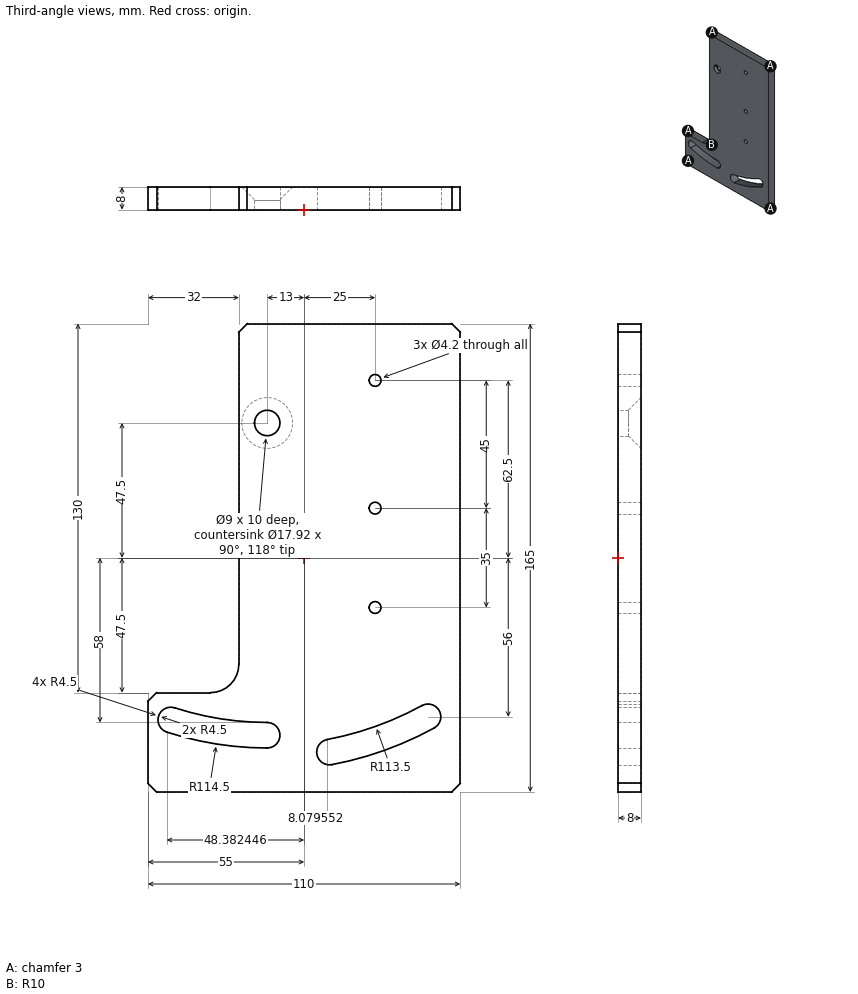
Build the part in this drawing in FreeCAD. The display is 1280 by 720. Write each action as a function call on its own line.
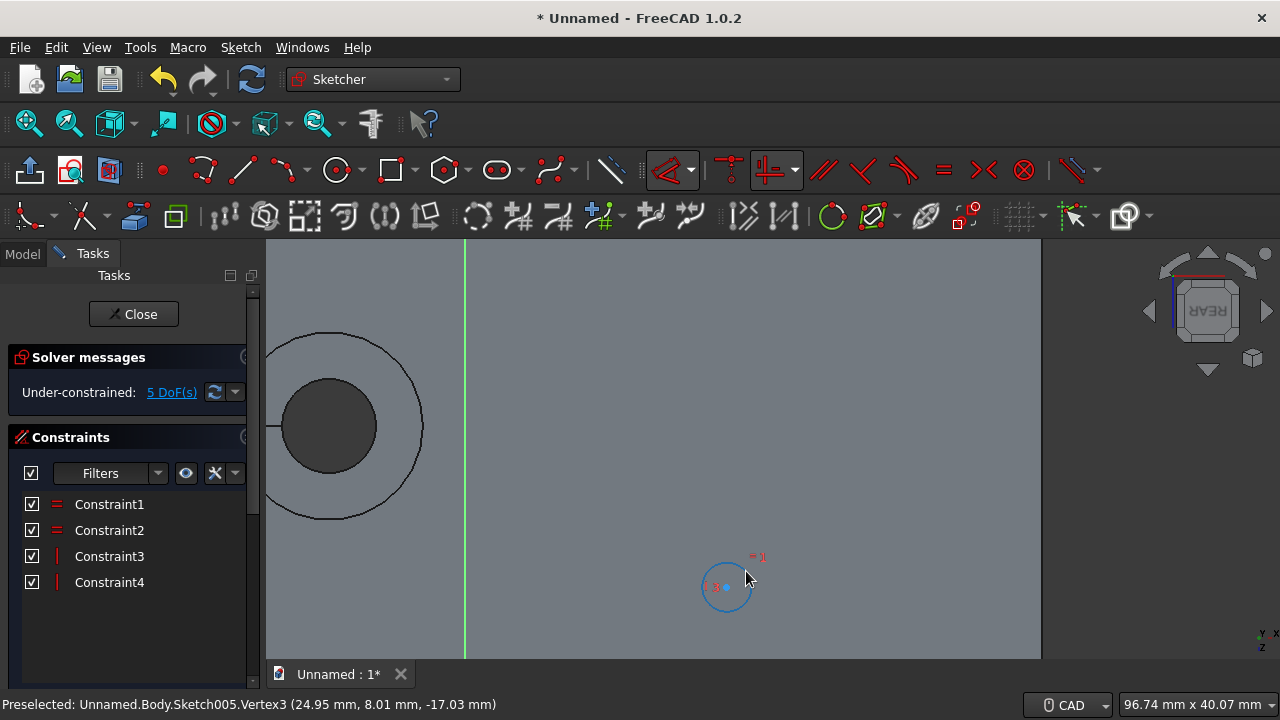
click(744, 570)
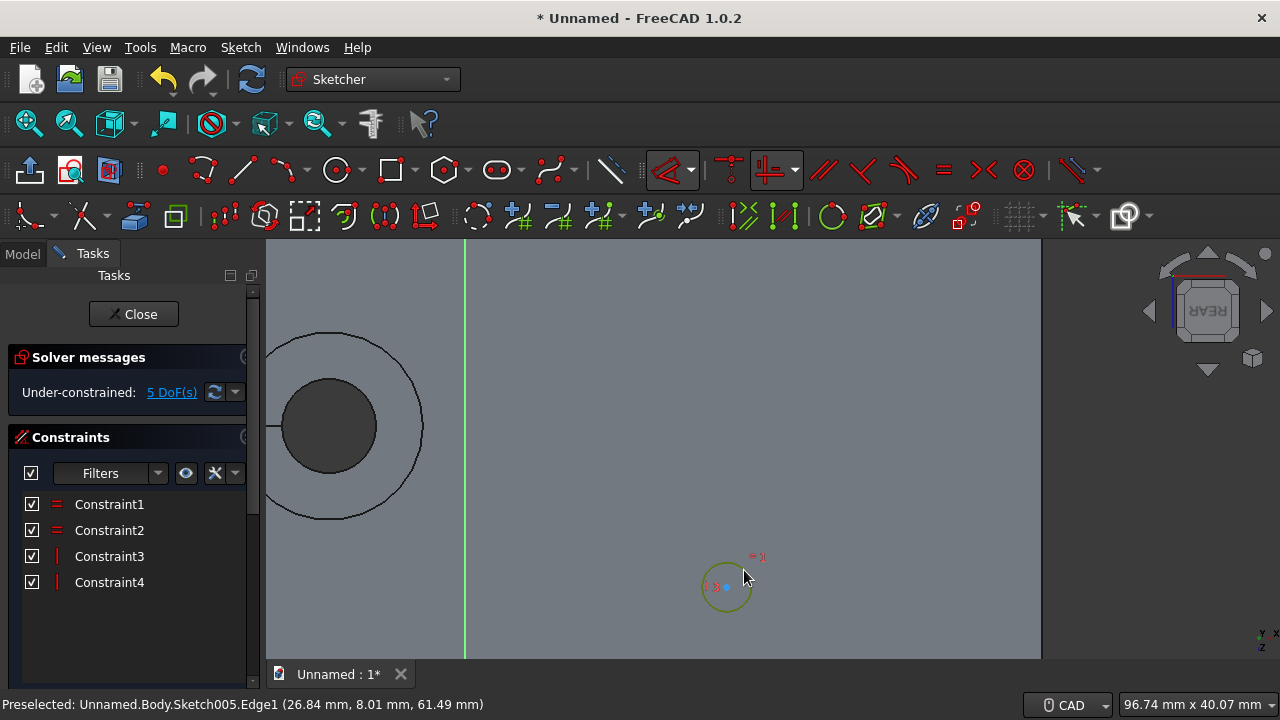
click(694, 170)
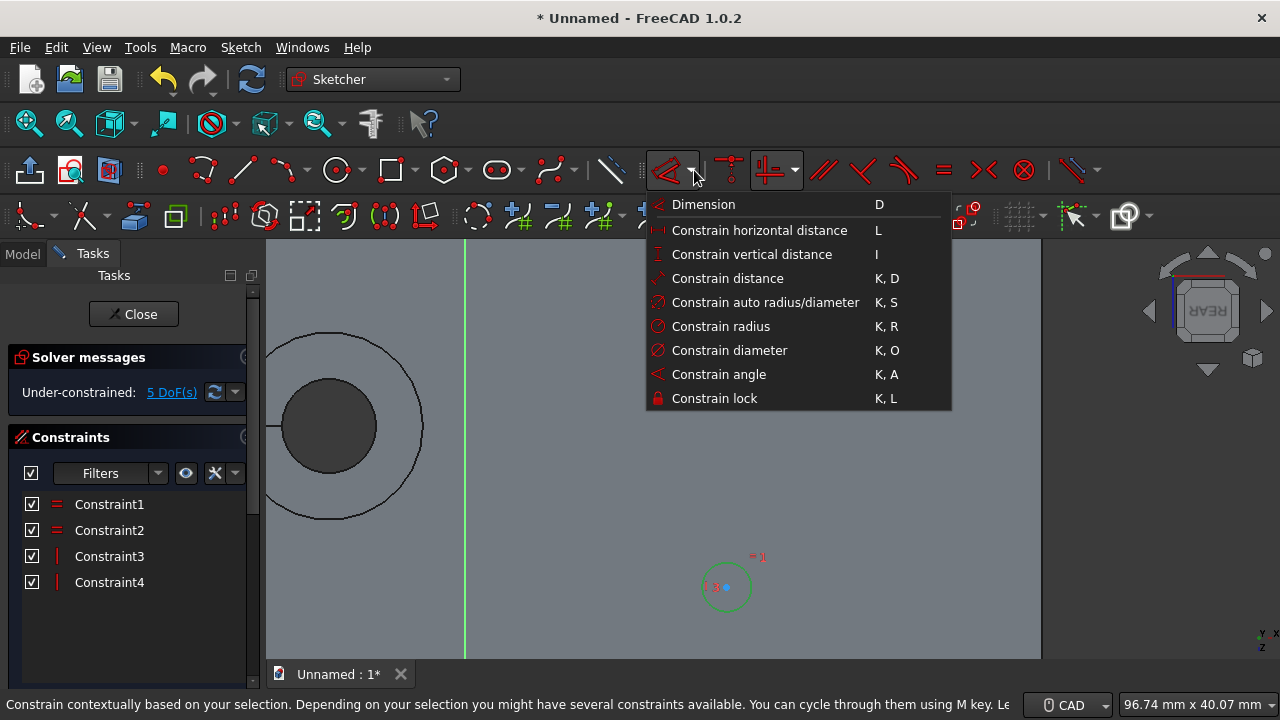
click(799, 350)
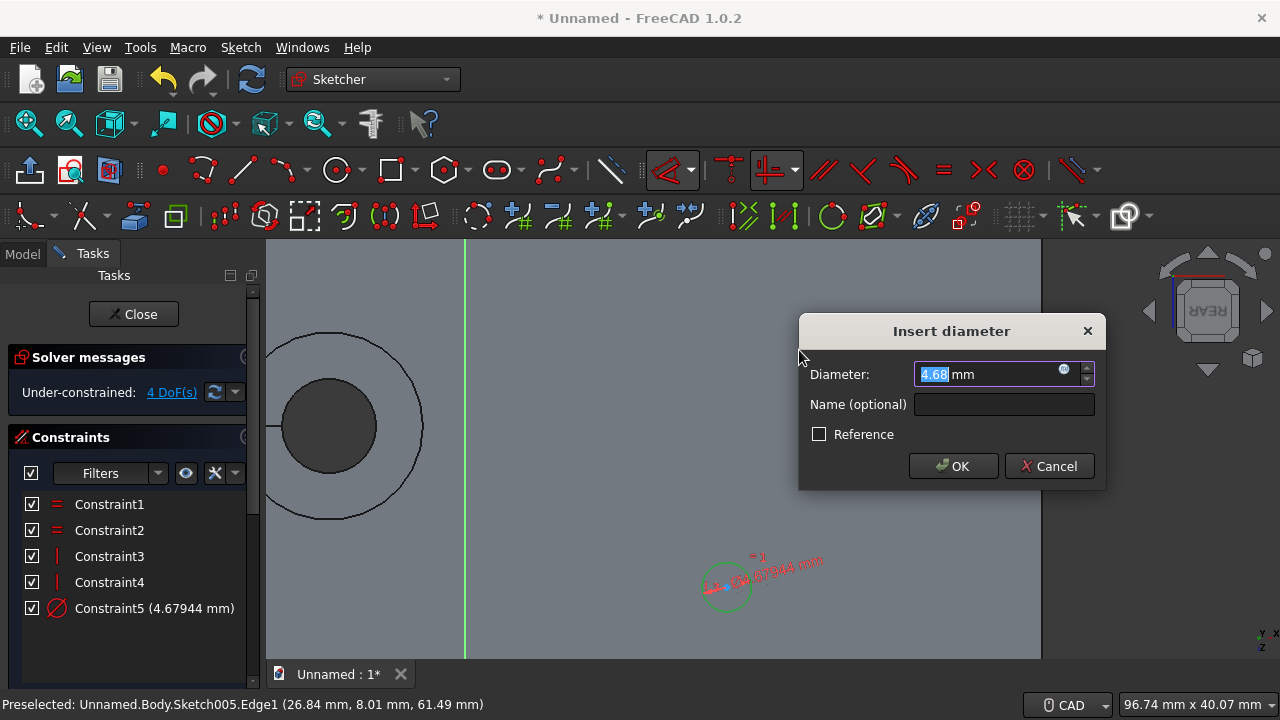
text(4.2)
key(Return)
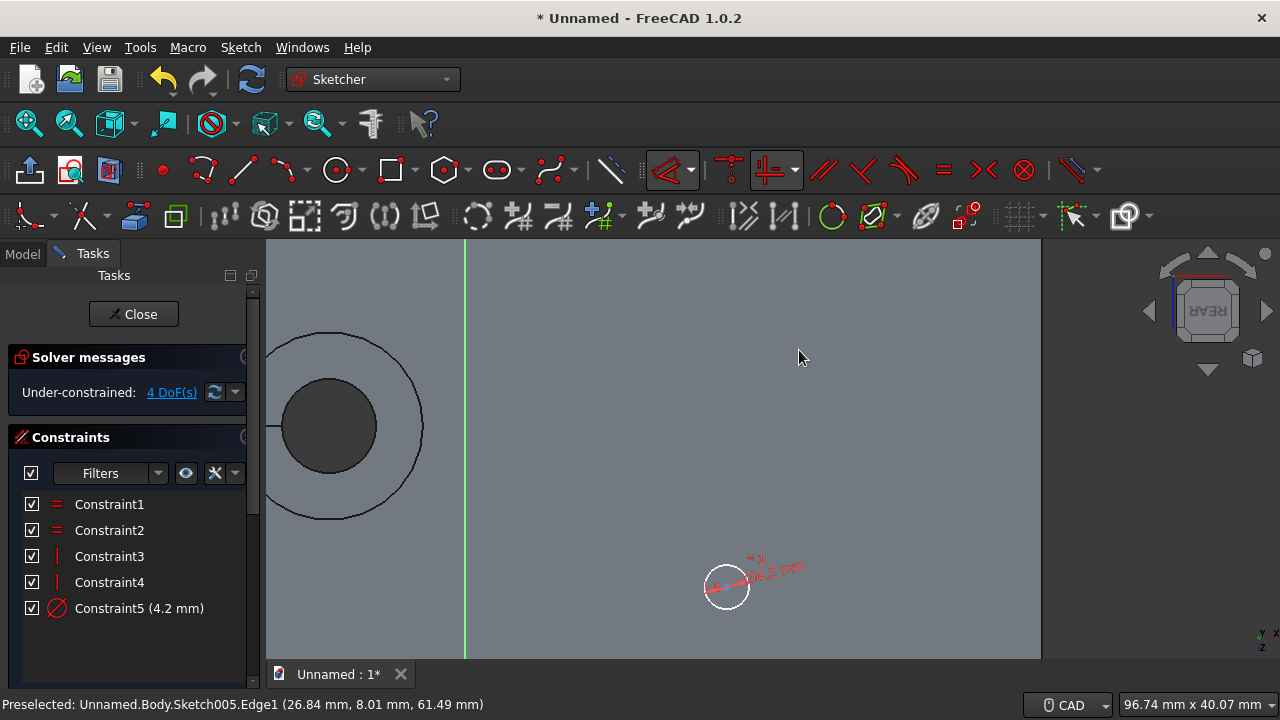
click(727, 587)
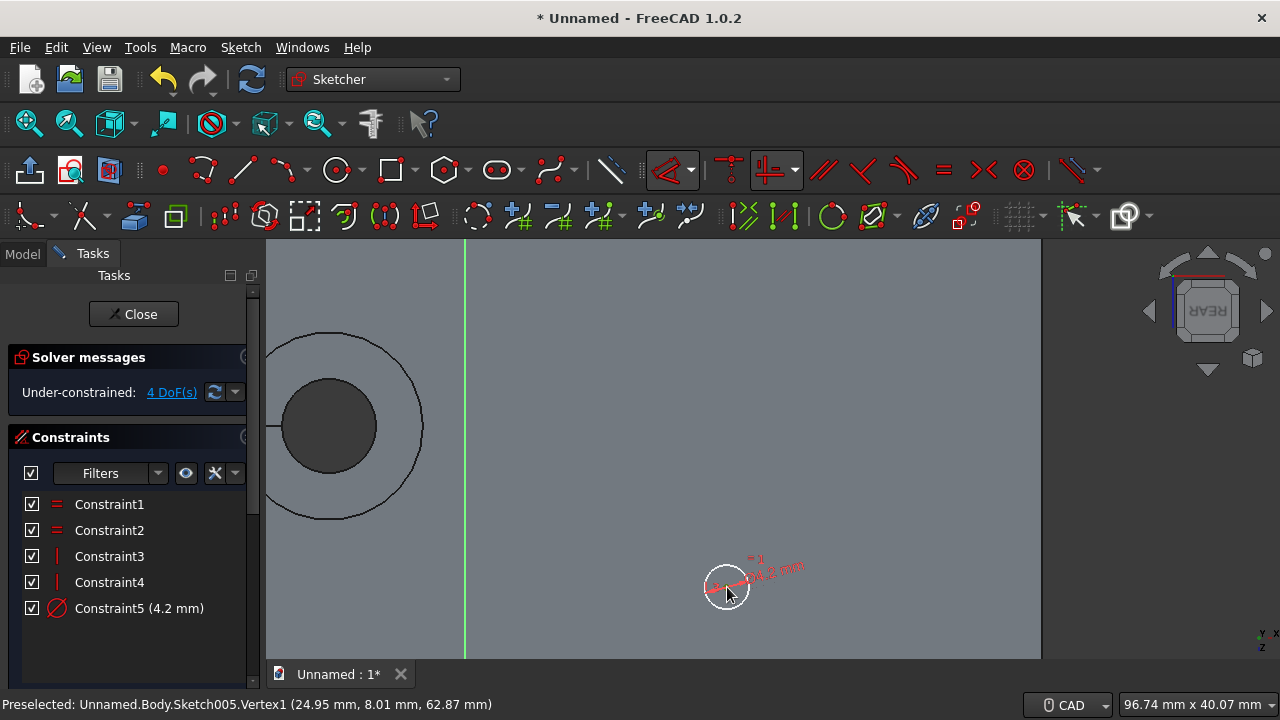
click(694, 170)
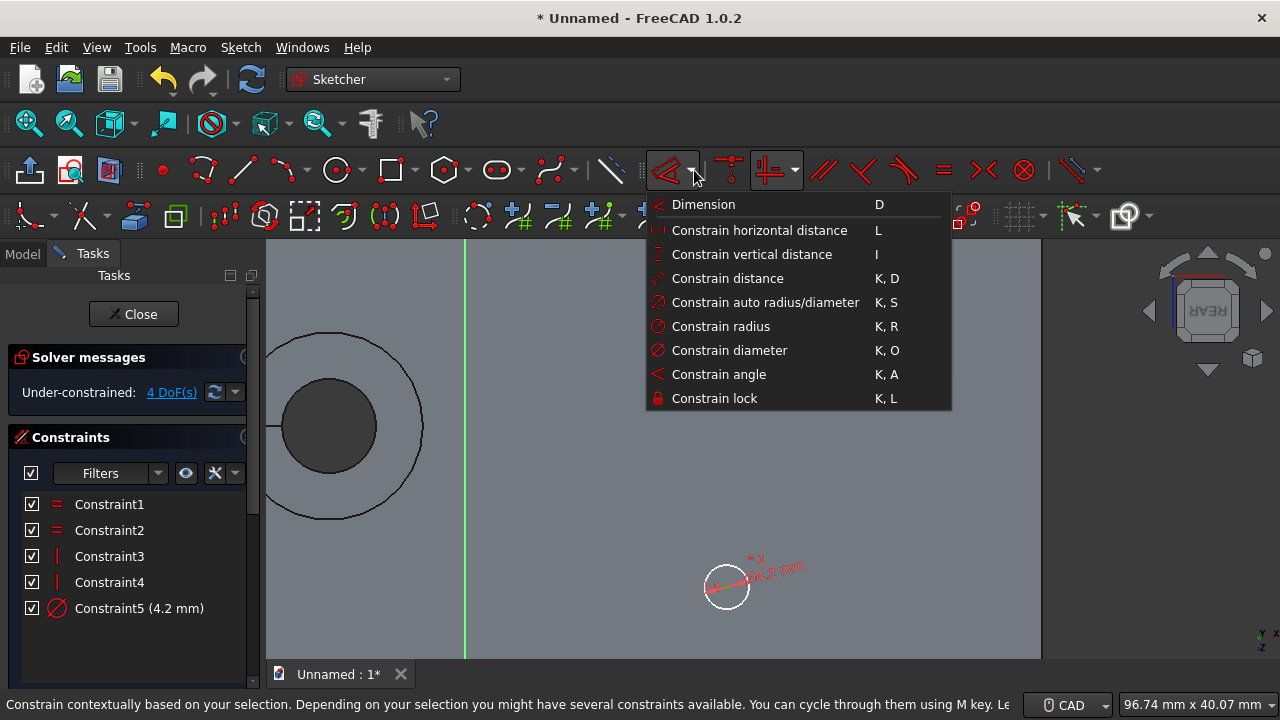
click(799, 230)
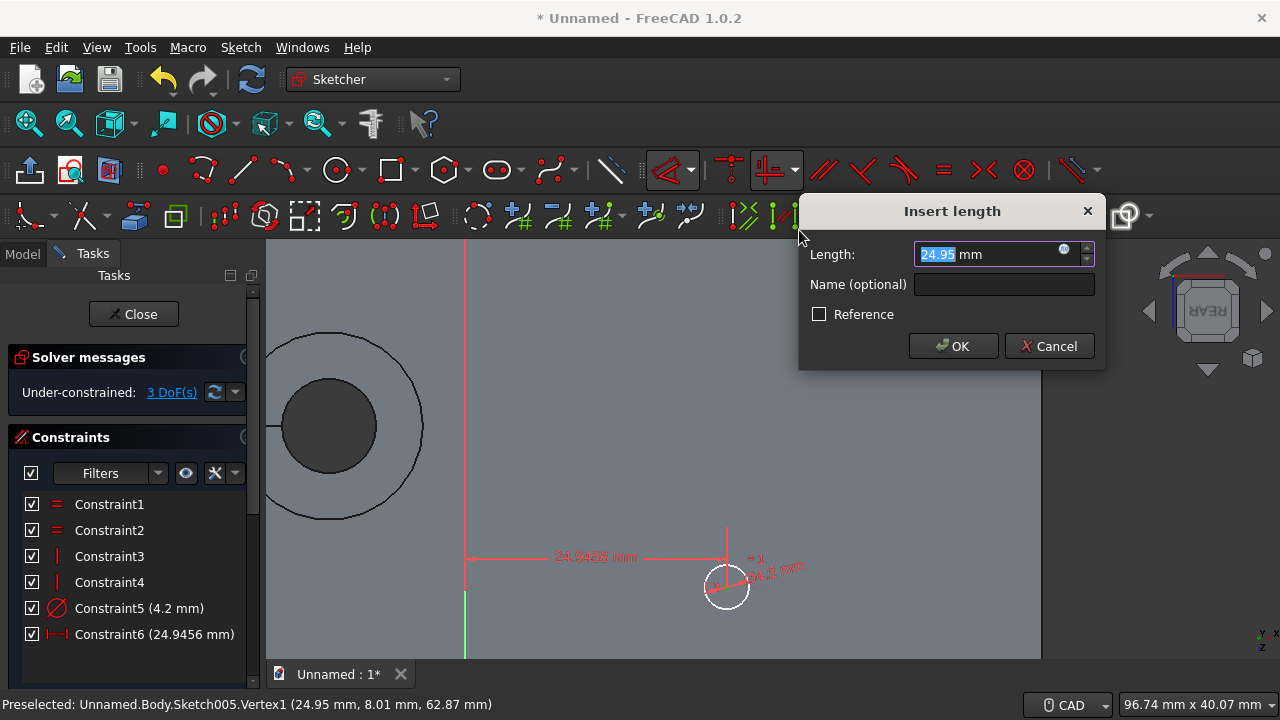
text(25)
key(Return)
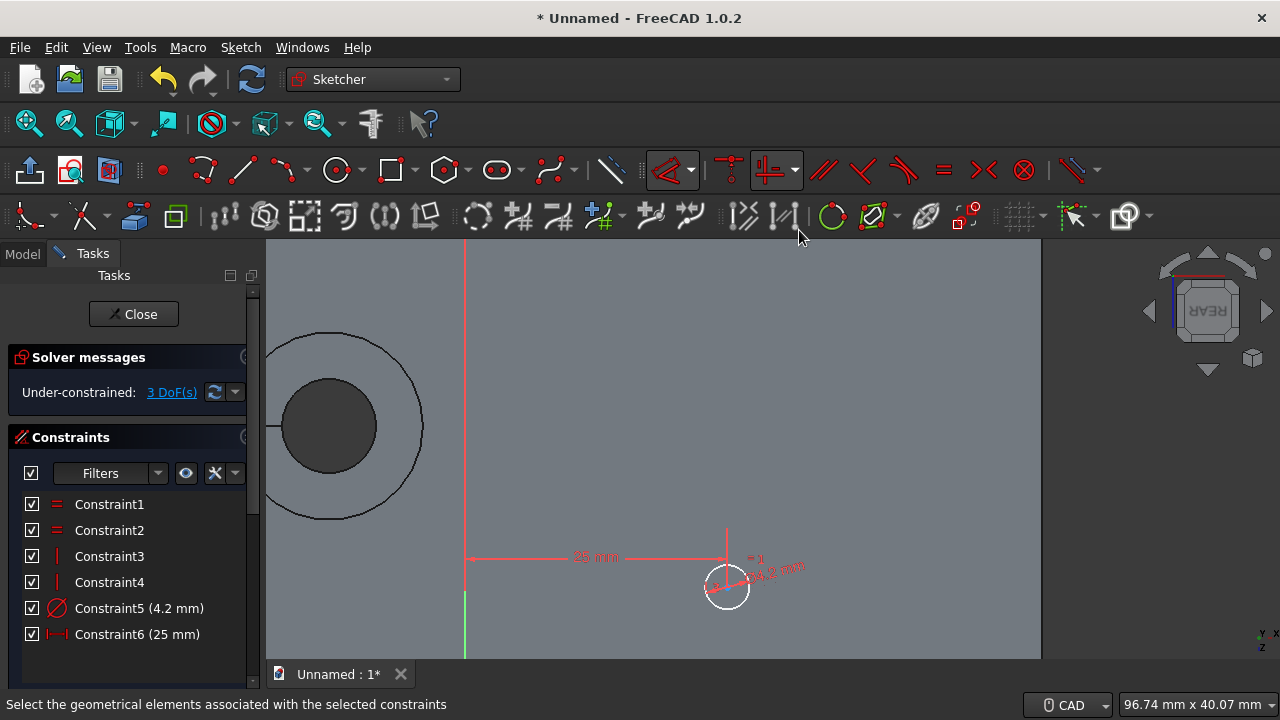
click(727, 587)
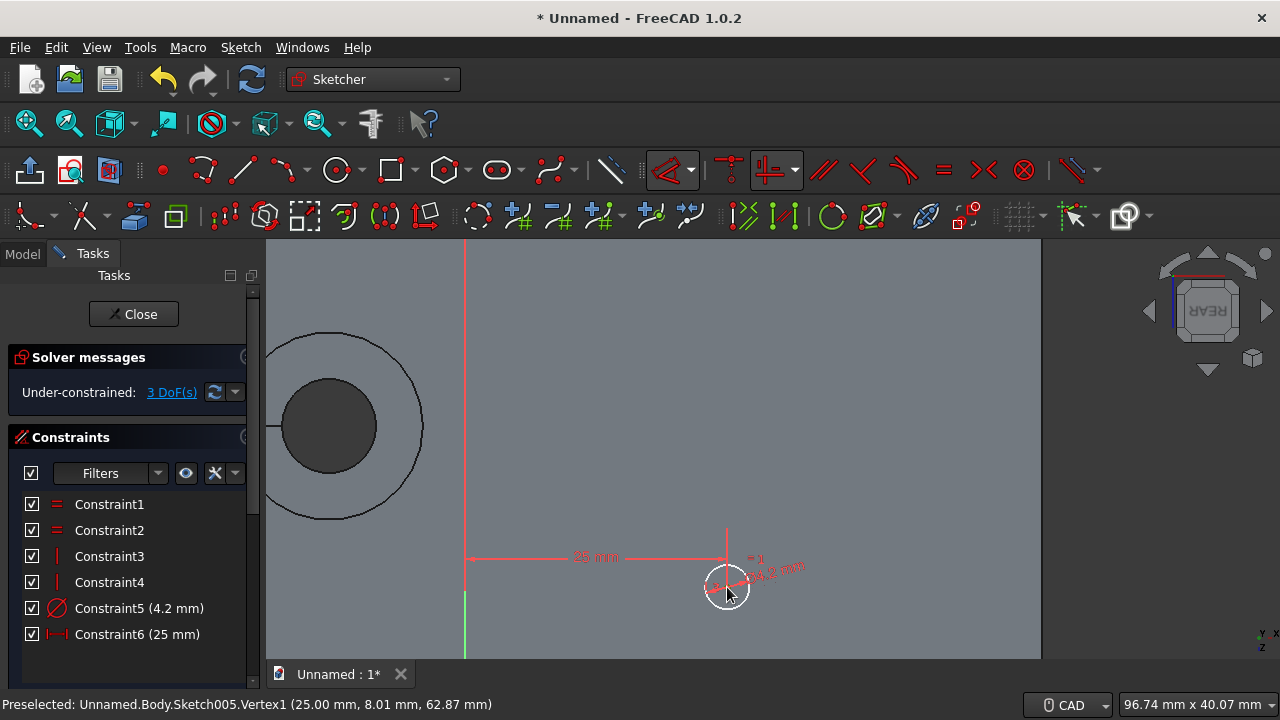
scroll(746, 572, down, 6)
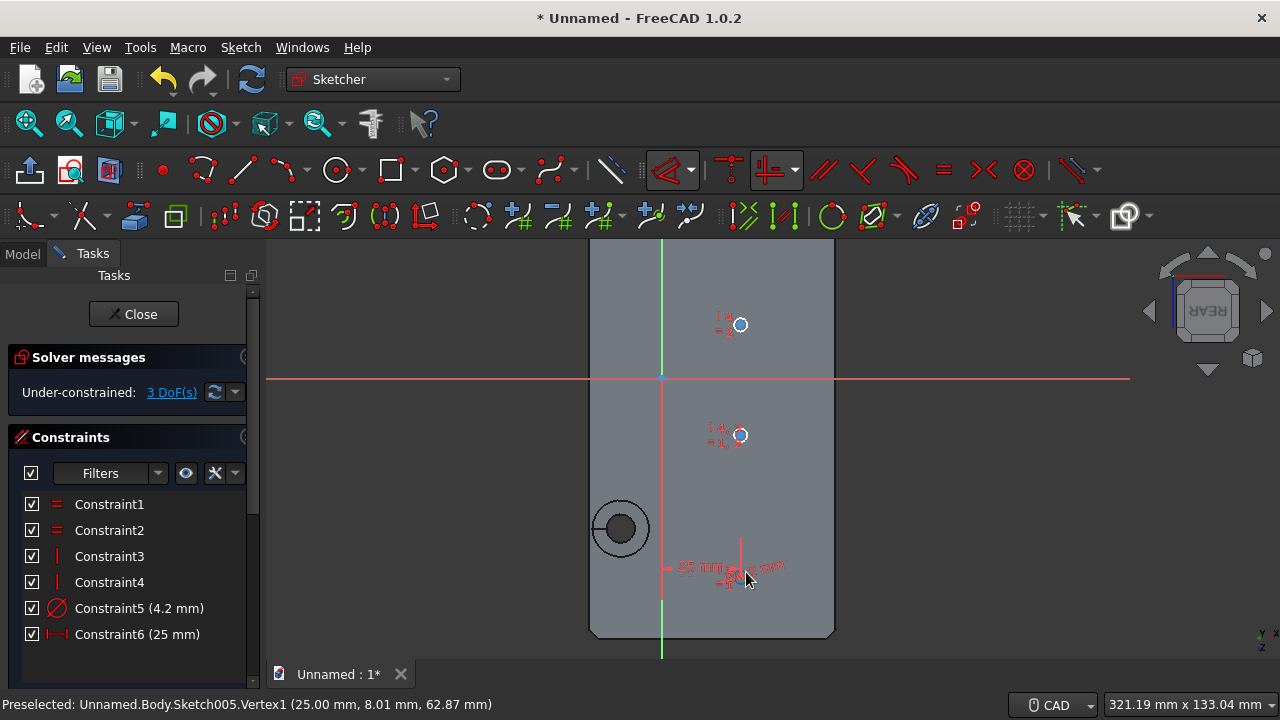
click(741, 435)